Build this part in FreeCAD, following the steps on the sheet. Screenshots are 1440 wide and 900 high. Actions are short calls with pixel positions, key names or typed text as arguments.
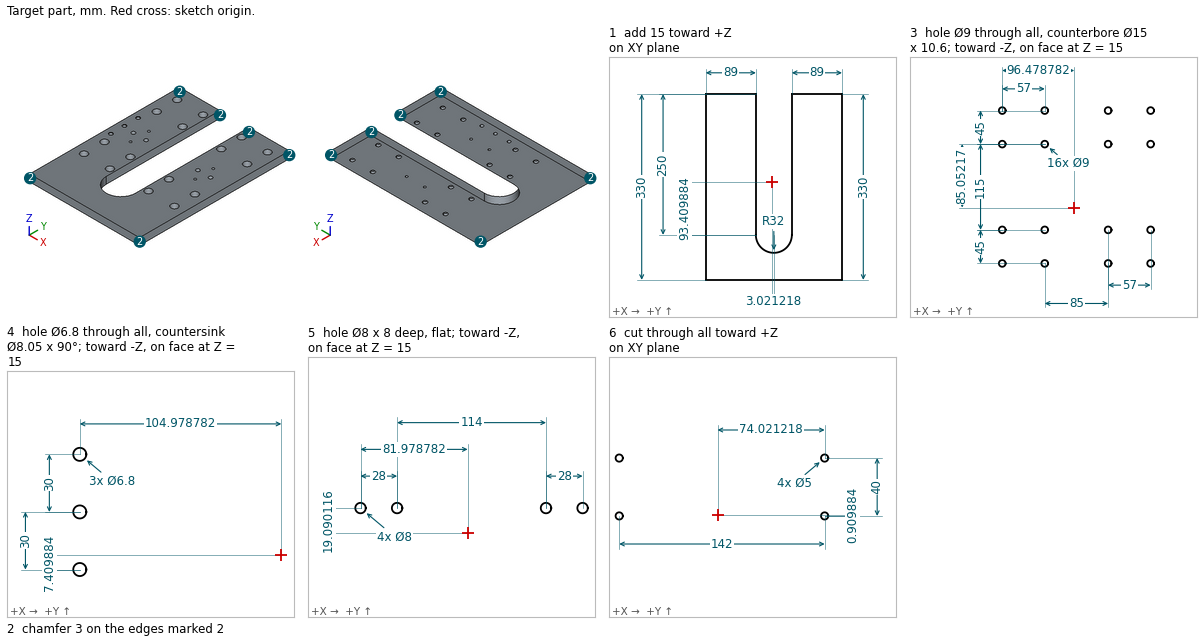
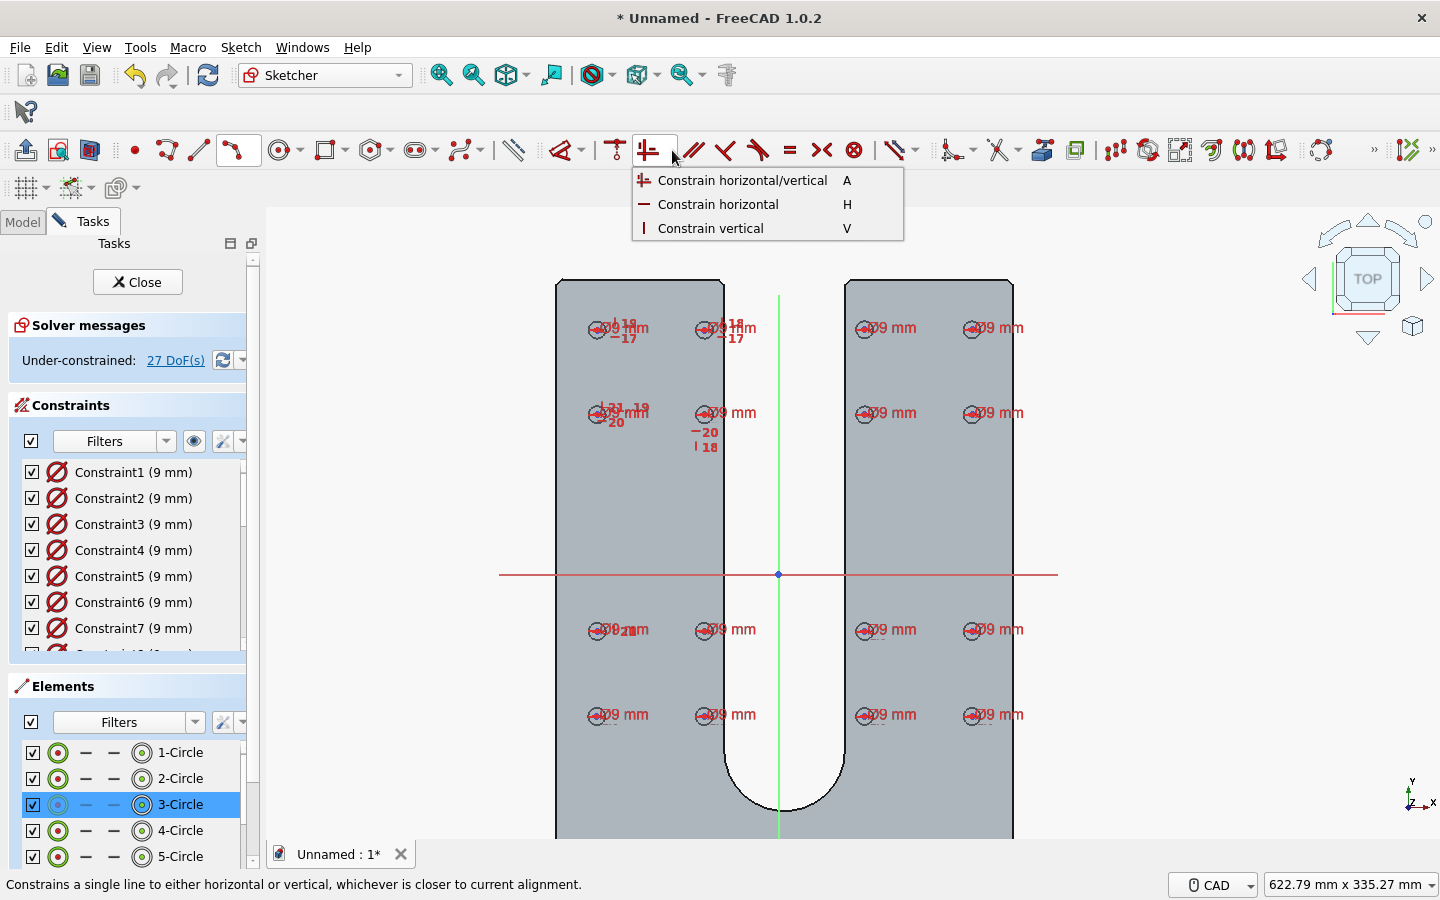
click(768, 228)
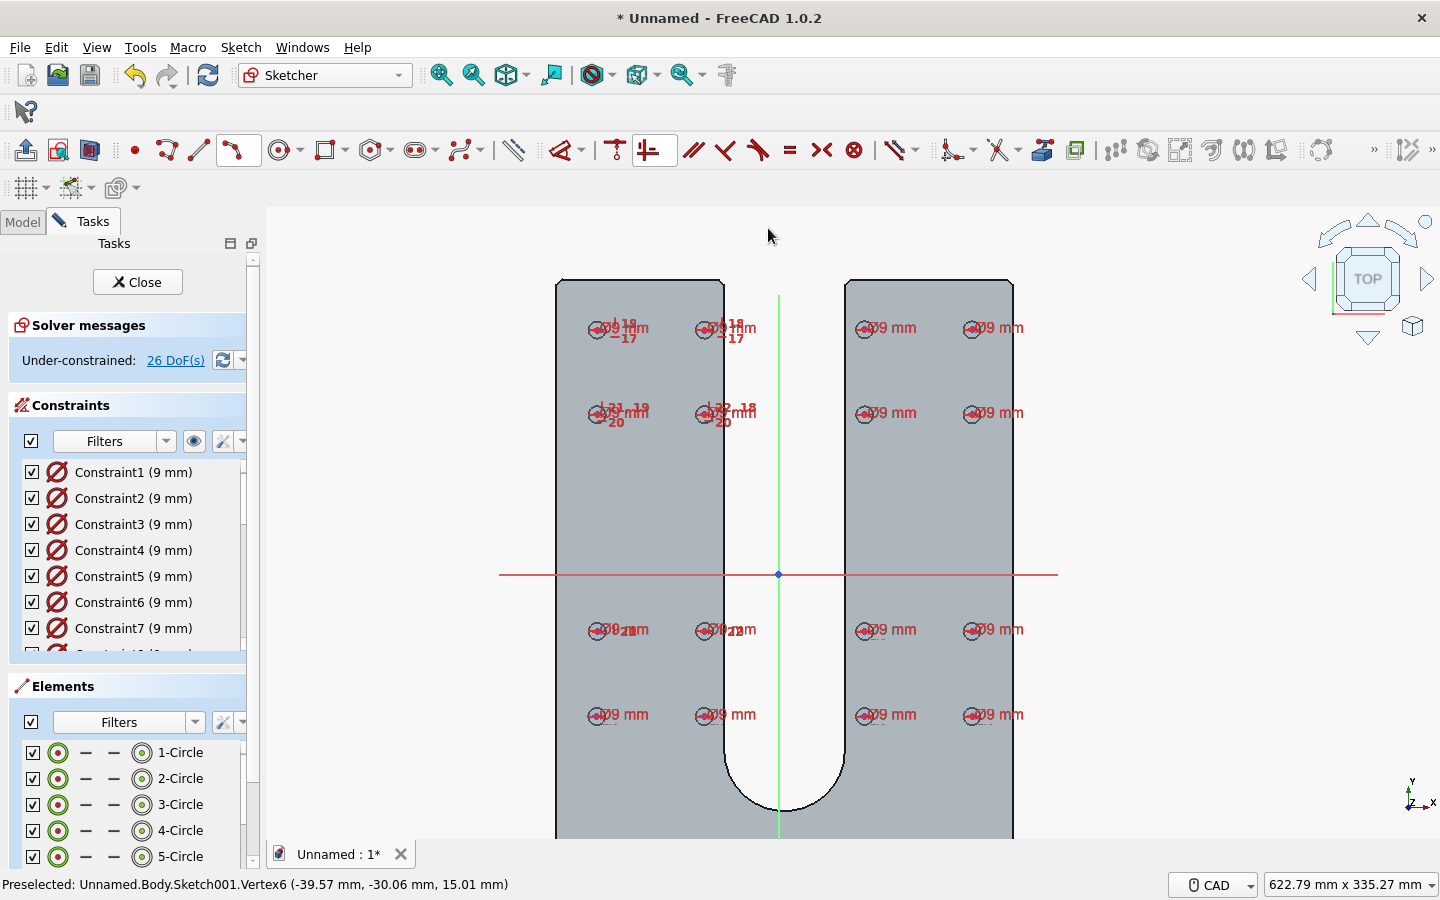
click(597, 631)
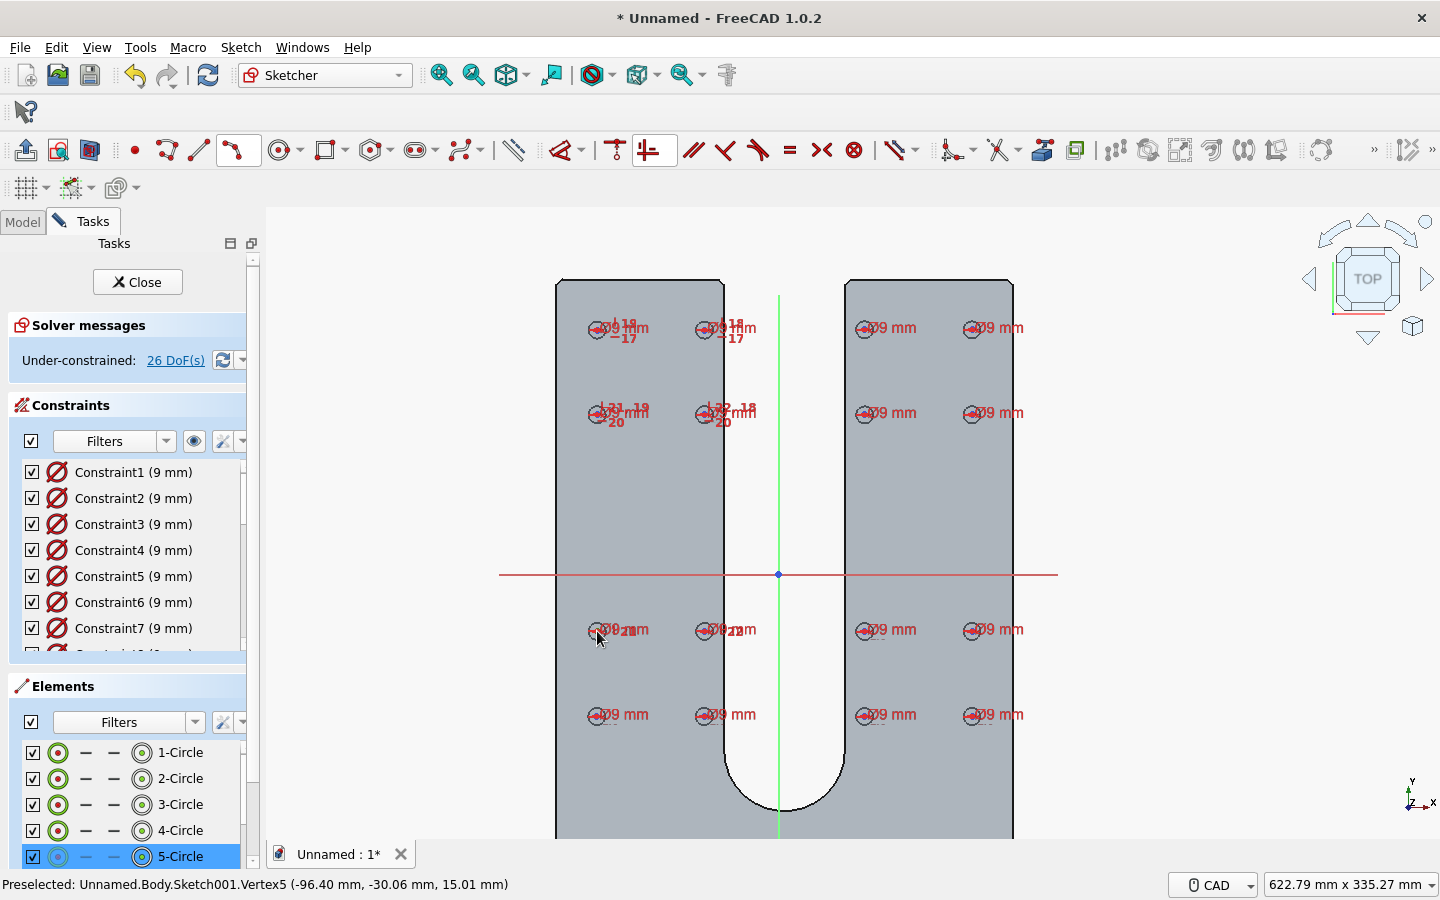
click(705, 631)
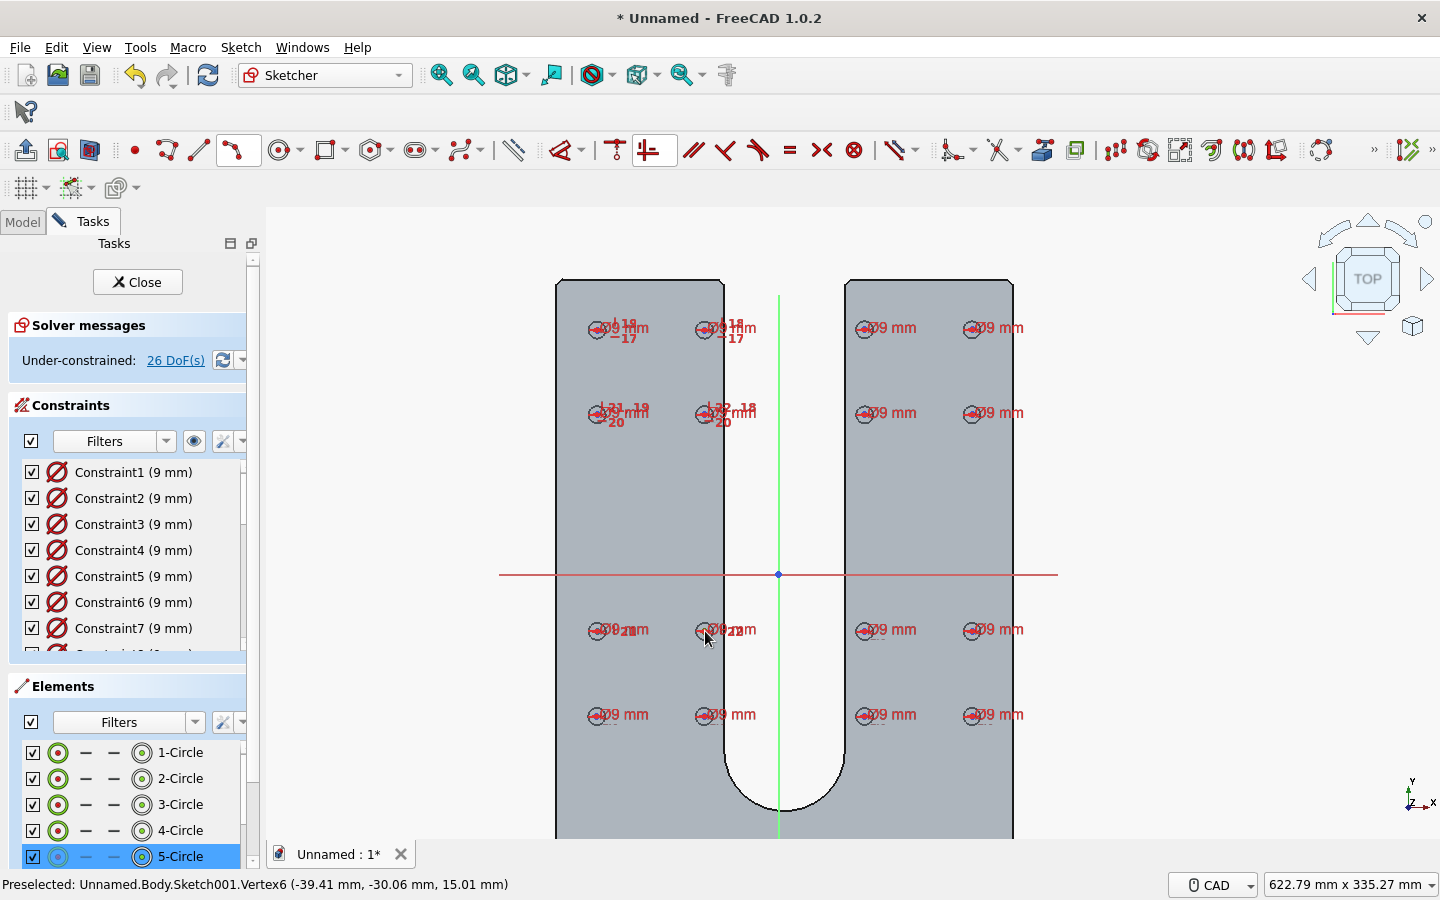
key(h)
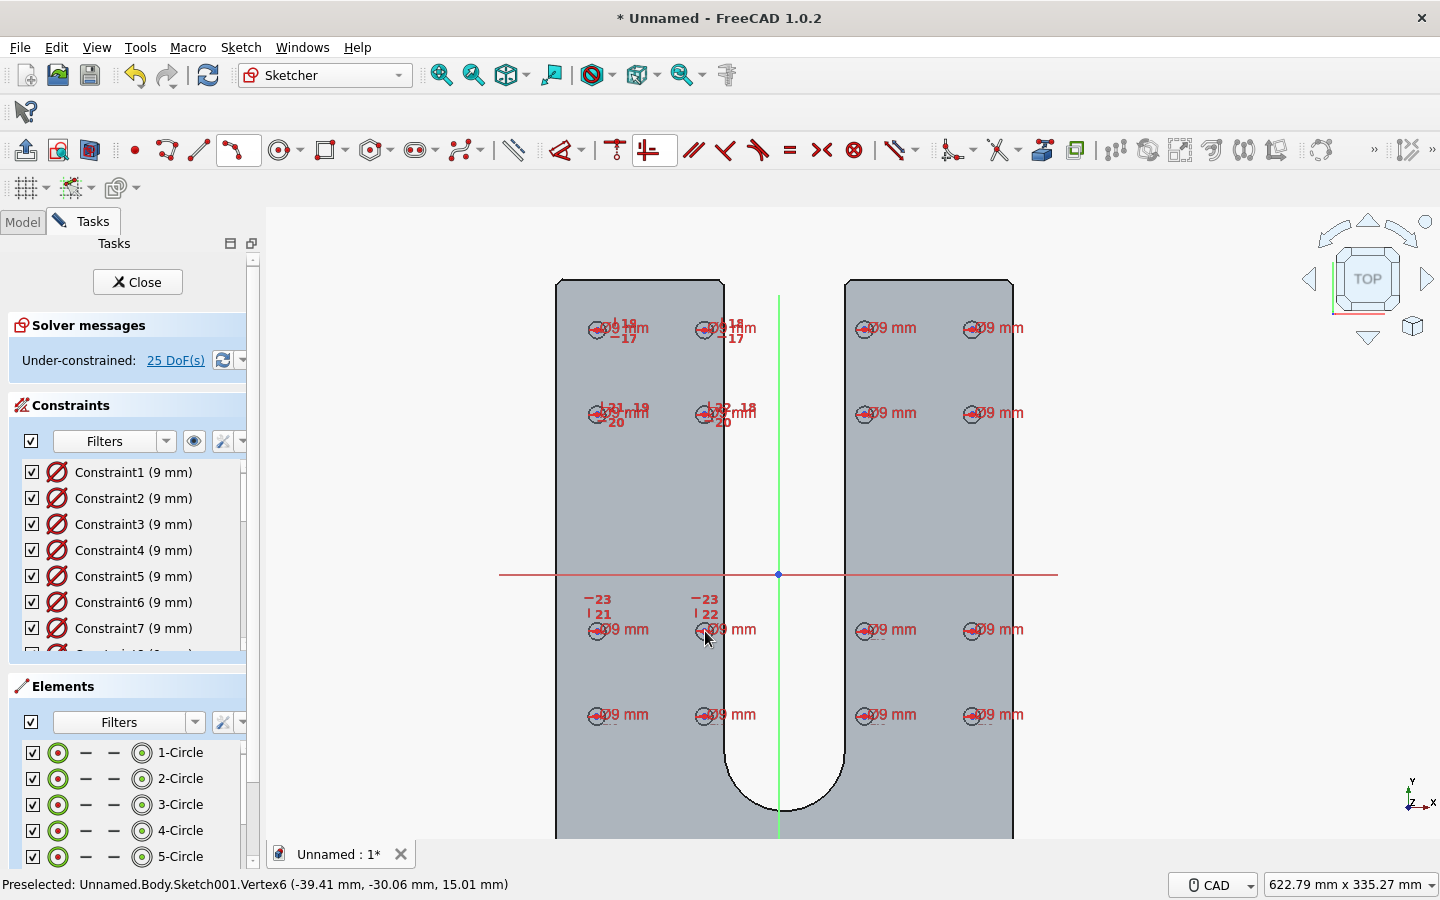
click(705, 631)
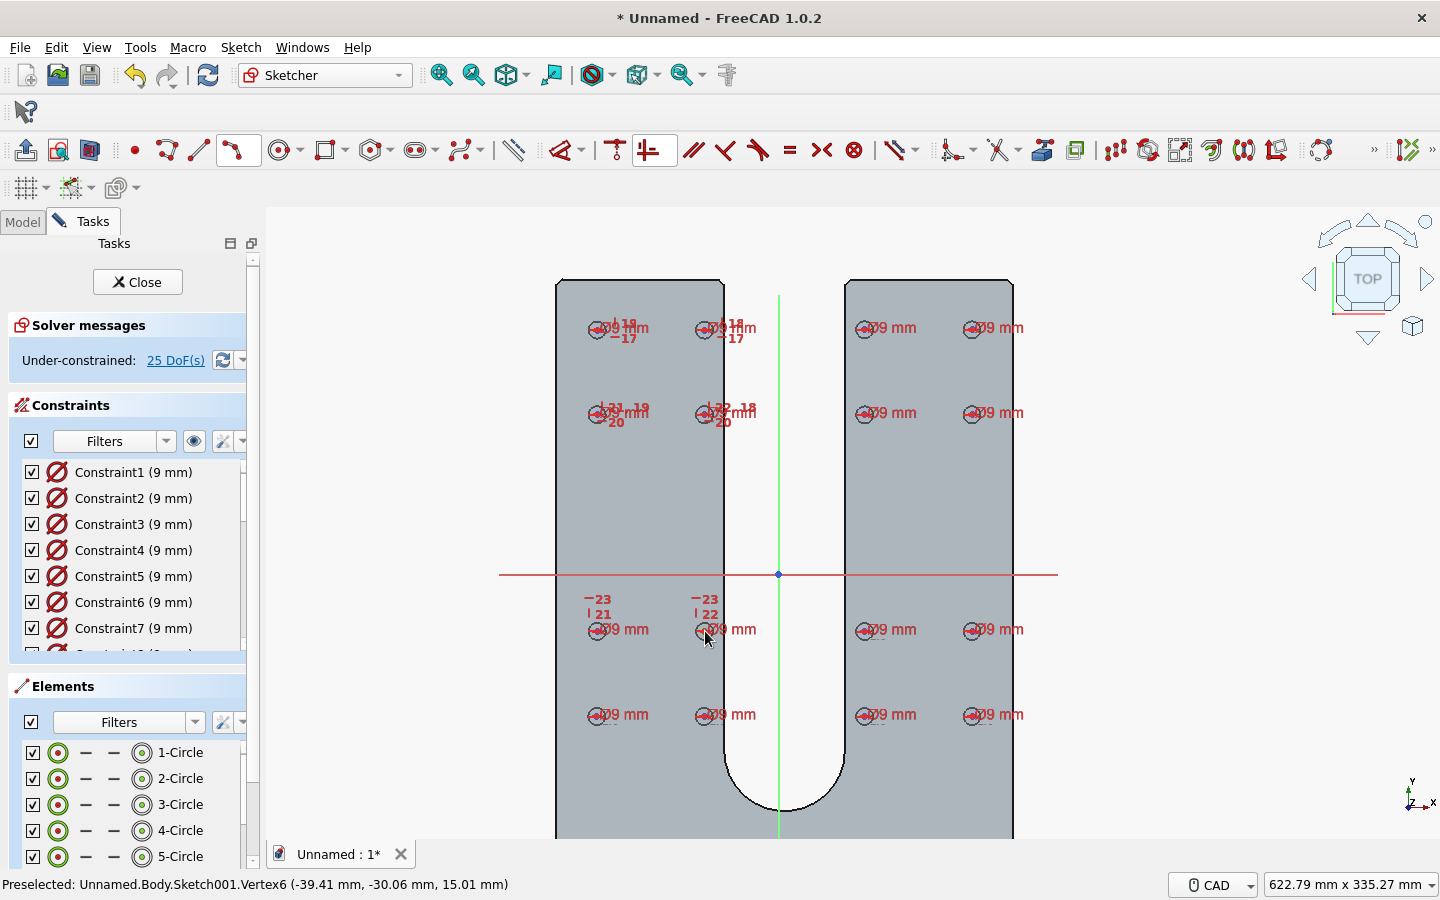
click(704, 717)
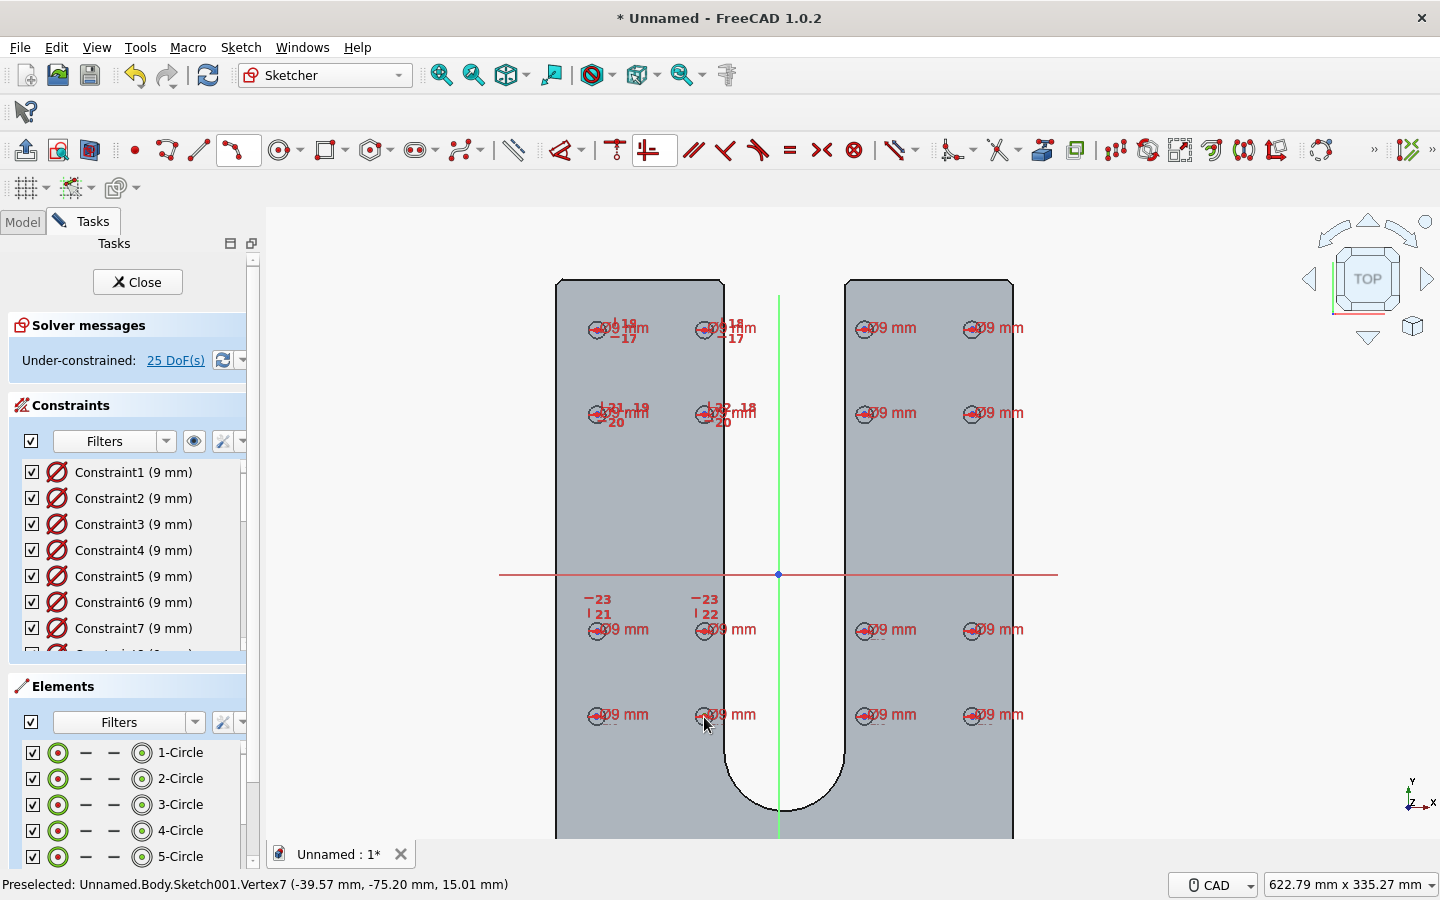
click(672, 150)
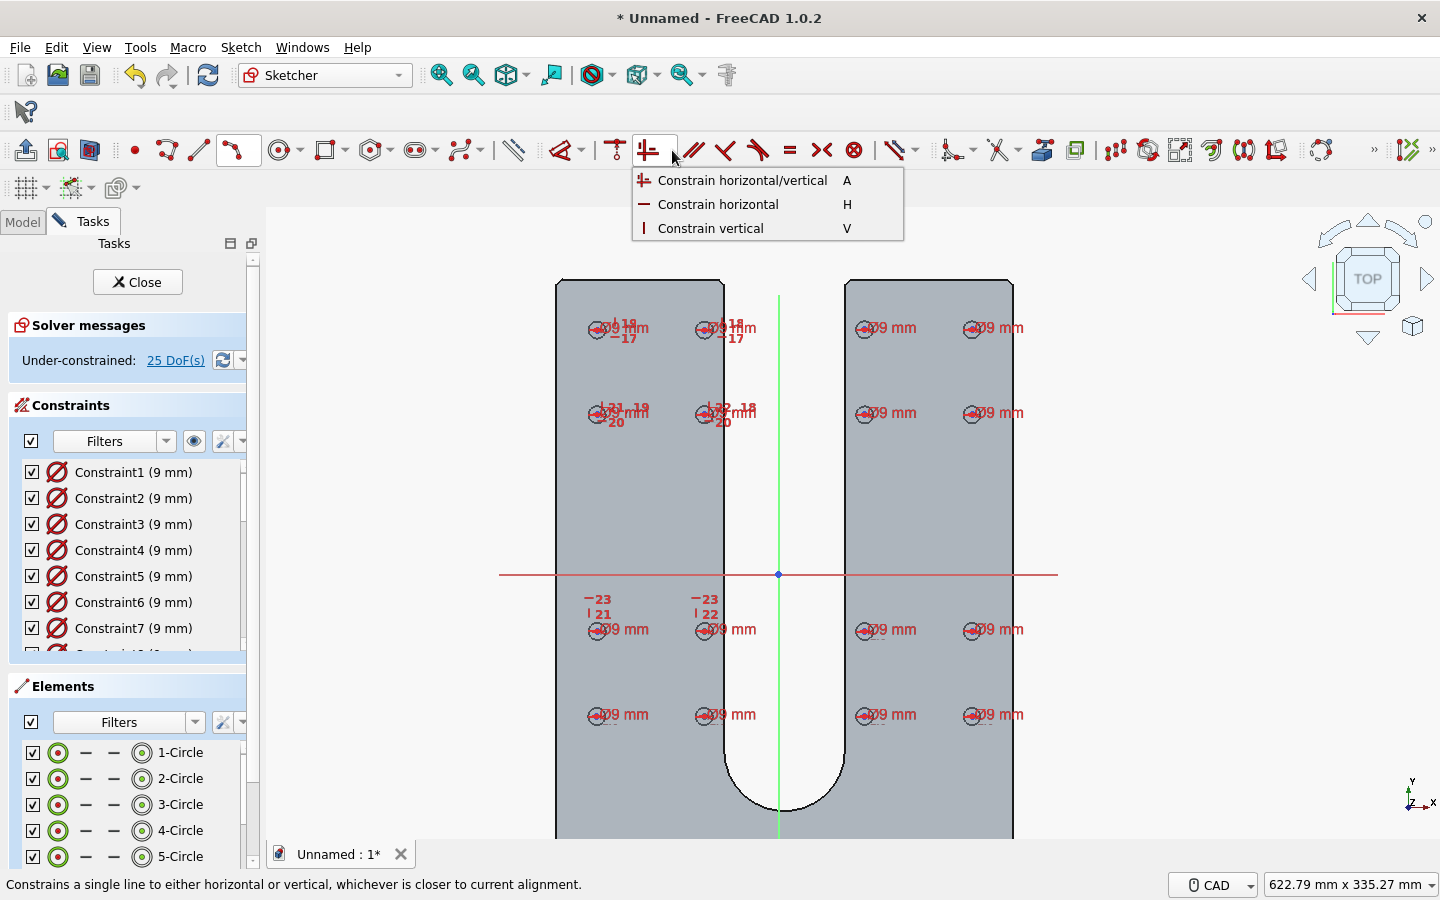
click(768, 228)